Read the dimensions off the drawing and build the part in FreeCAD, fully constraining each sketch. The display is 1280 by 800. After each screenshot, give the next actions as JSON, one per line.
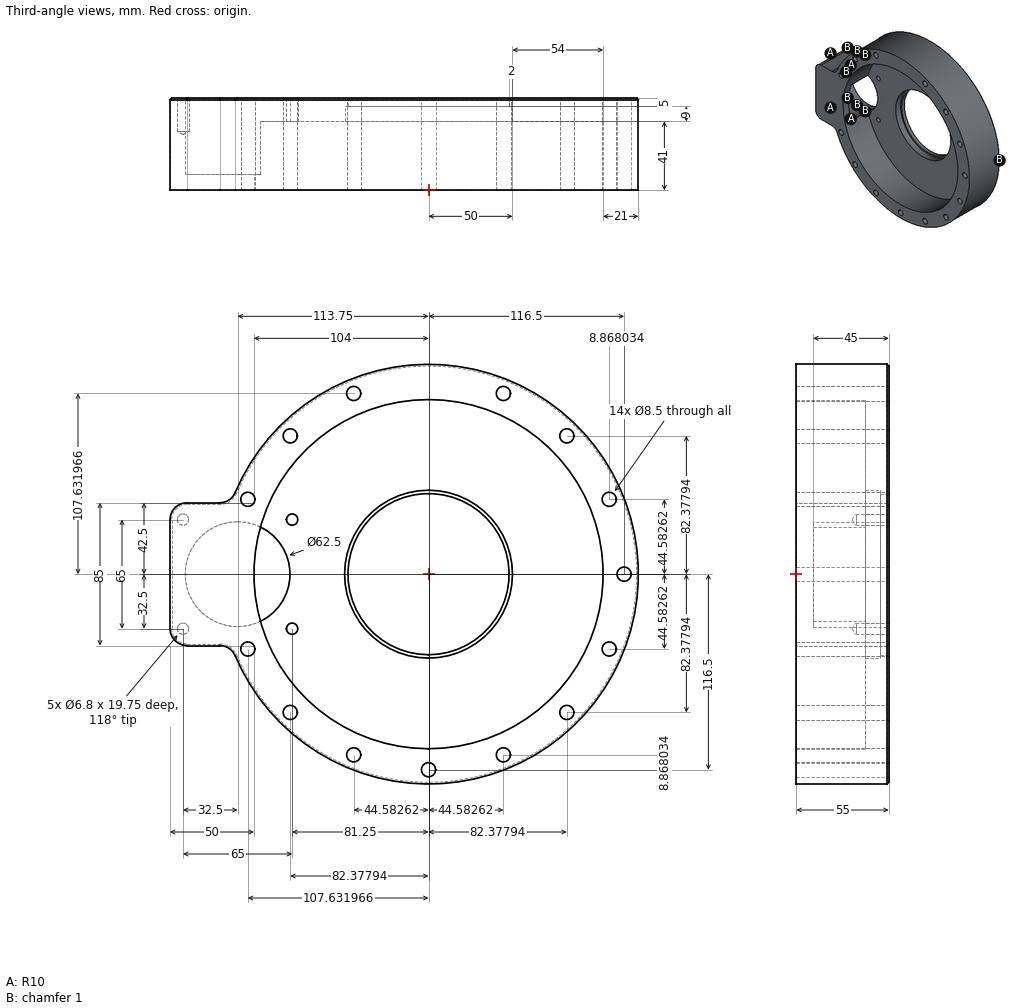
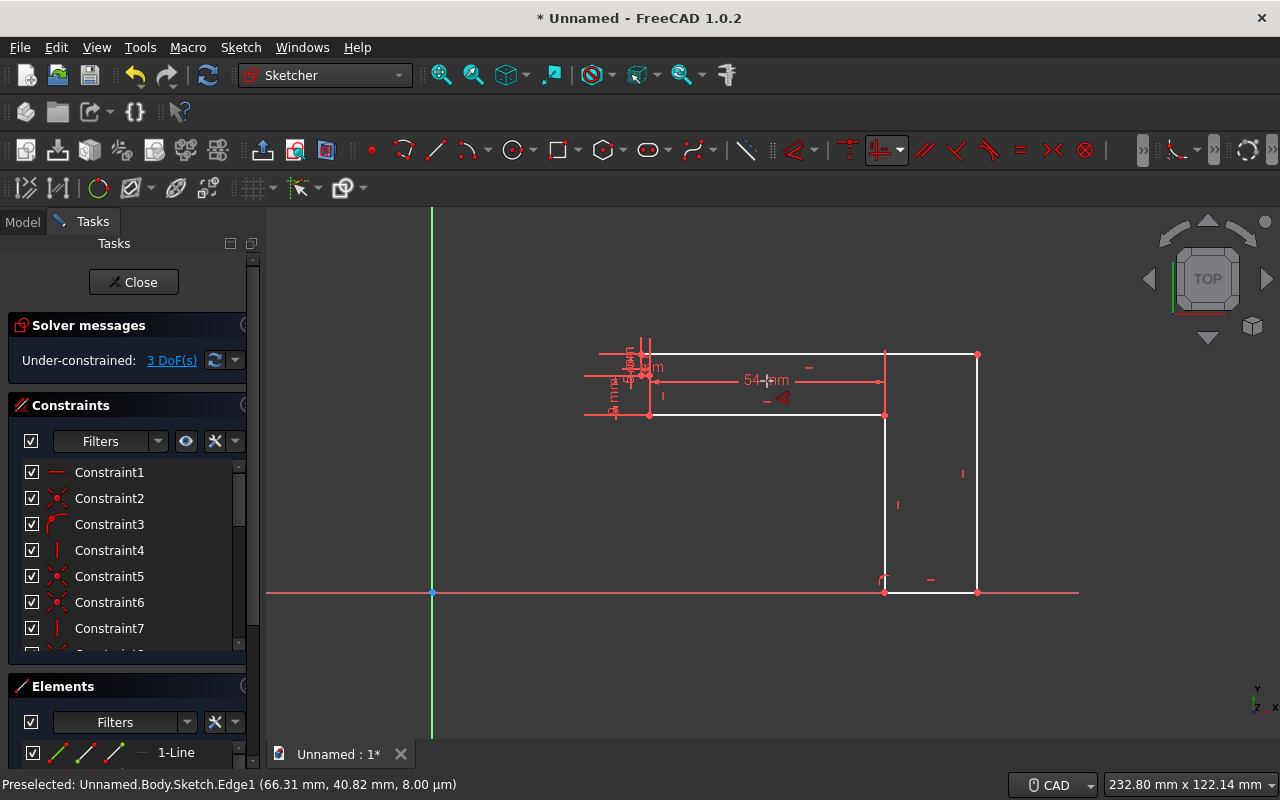
{"action": "left_click", "coordinate": [885, 468]}
{"action": "left_click", "coordinate": [919, 504]}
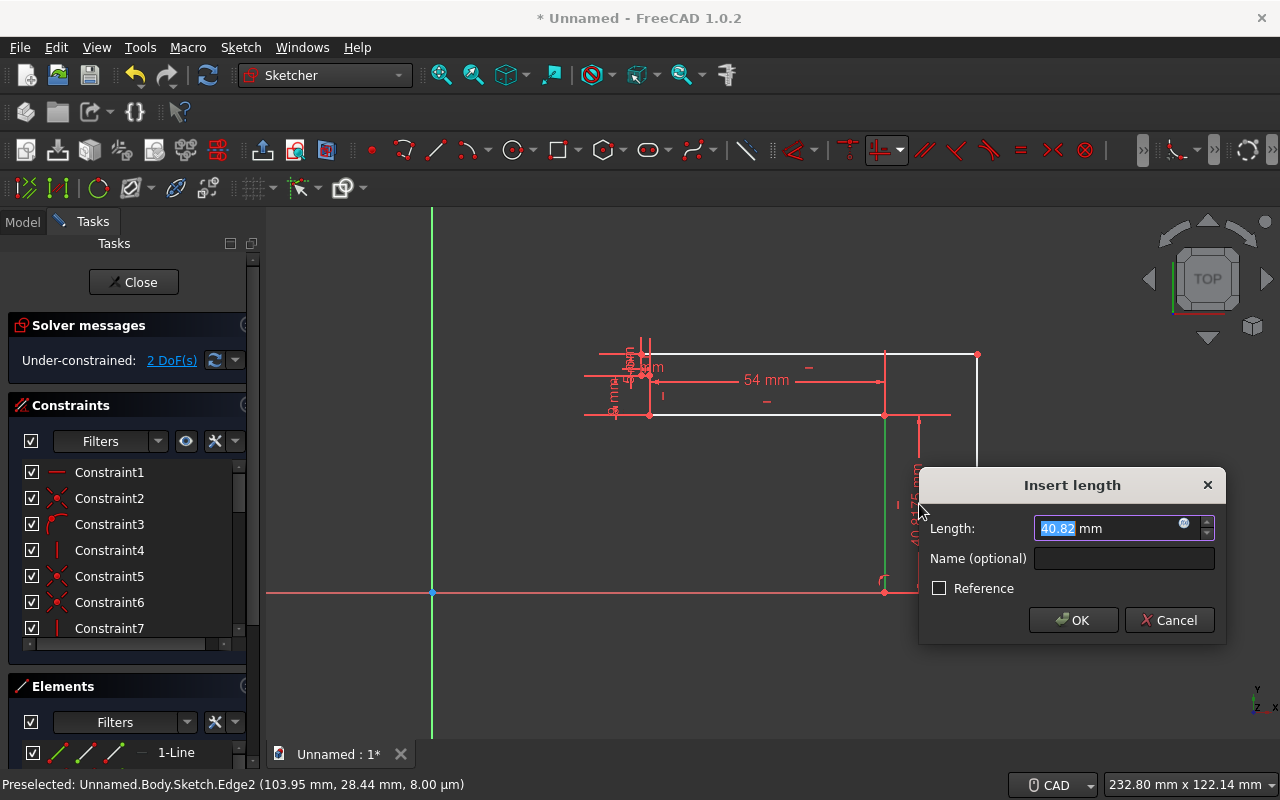
{"action": "type", "text": "41"}
{"action": "key", "text": "Return"}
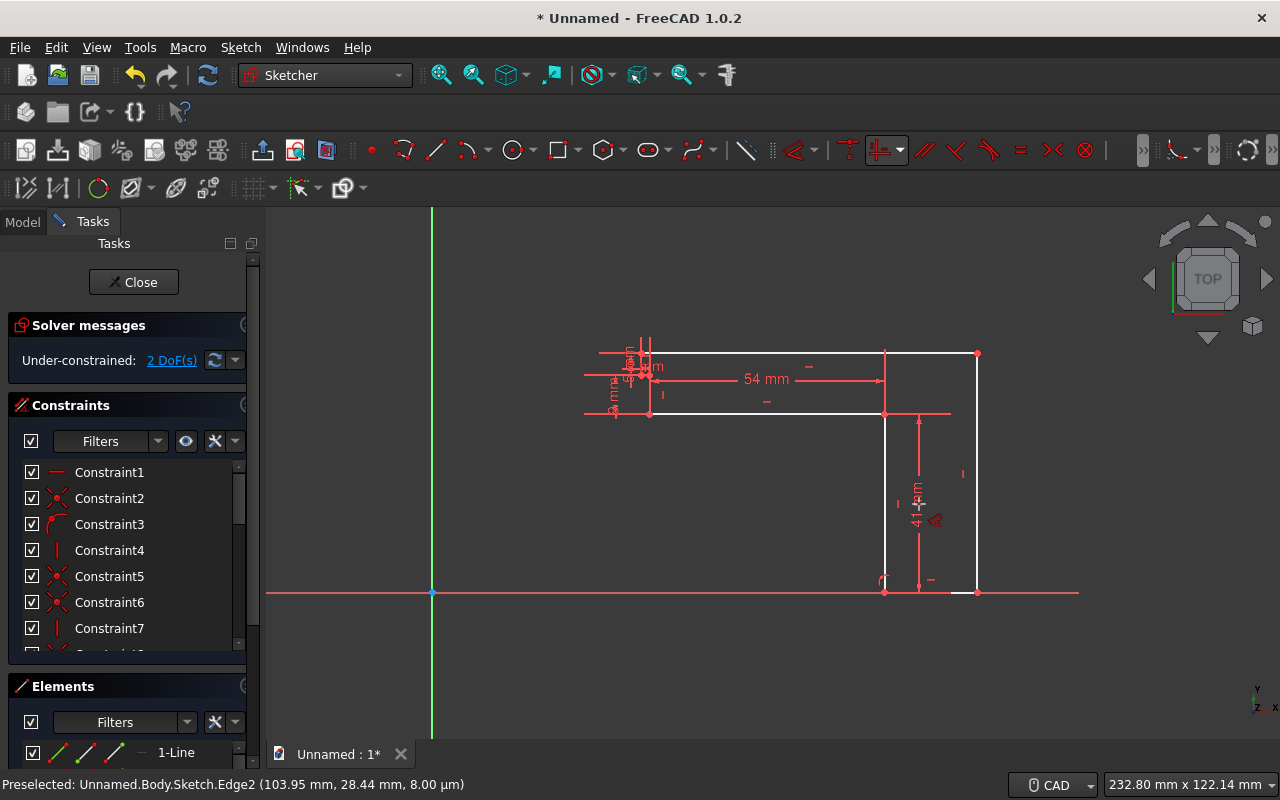
{"action": "left_click", "coordinate": [913, 593]}
{"action": "left_click", "coordinate": [931, 627]}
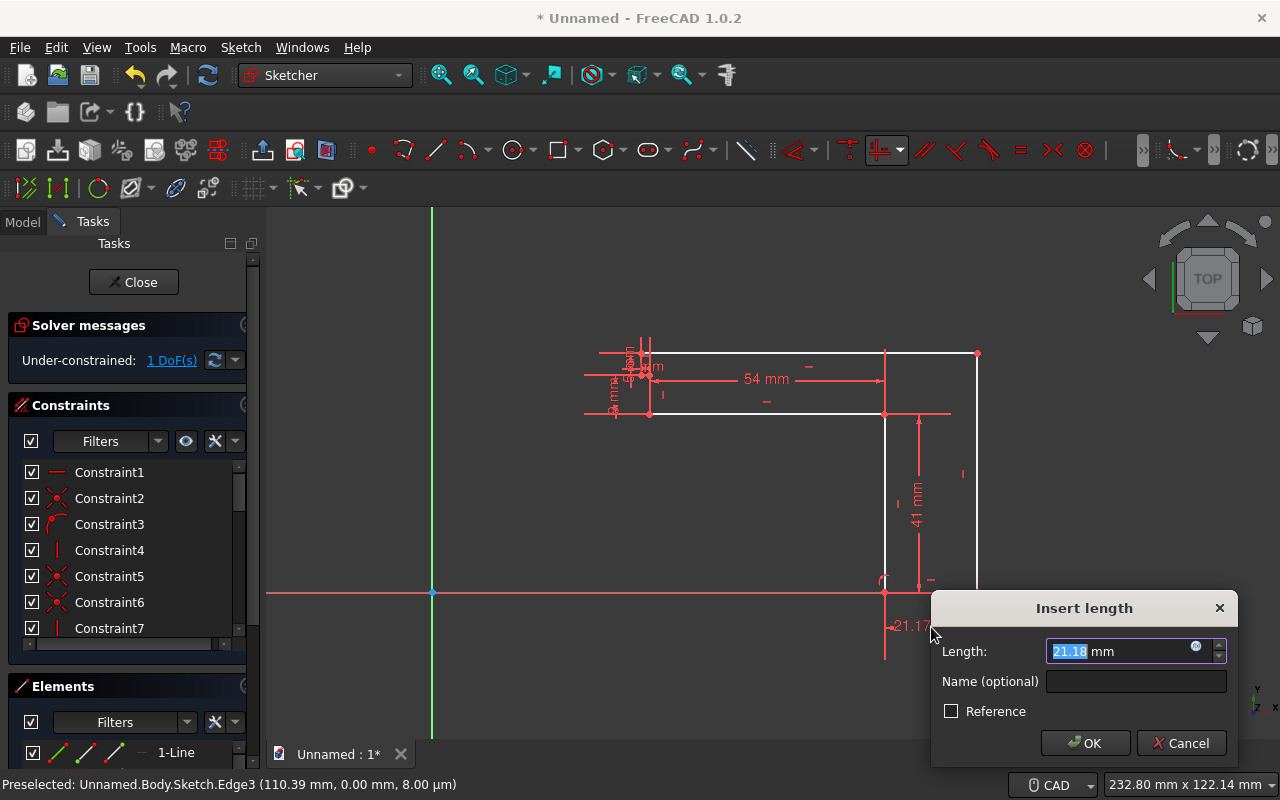
{"action": "type", "text": "21"}
{"action": "key", "text": "Return"}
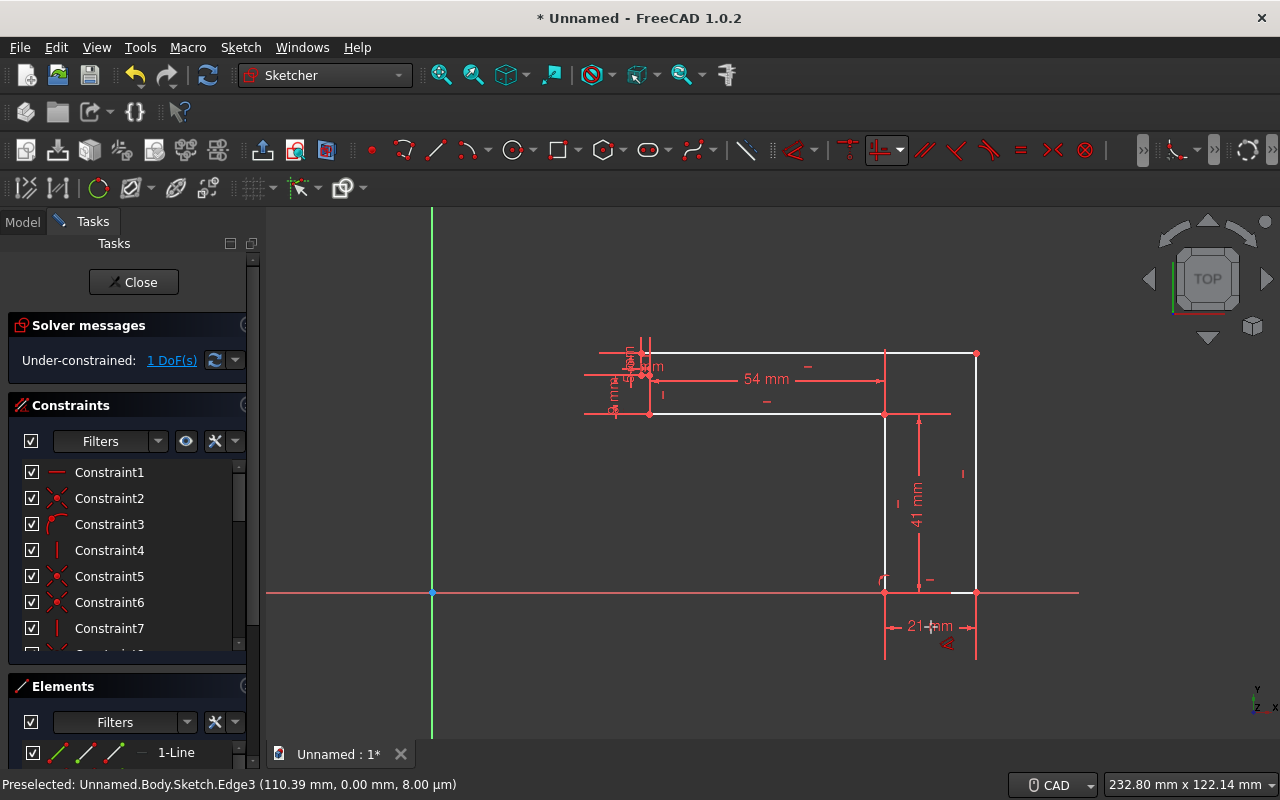
{"action": "left_click", "coordinate": [650, 414]}
{"action": "left_click", "coordinate": [541, 627]}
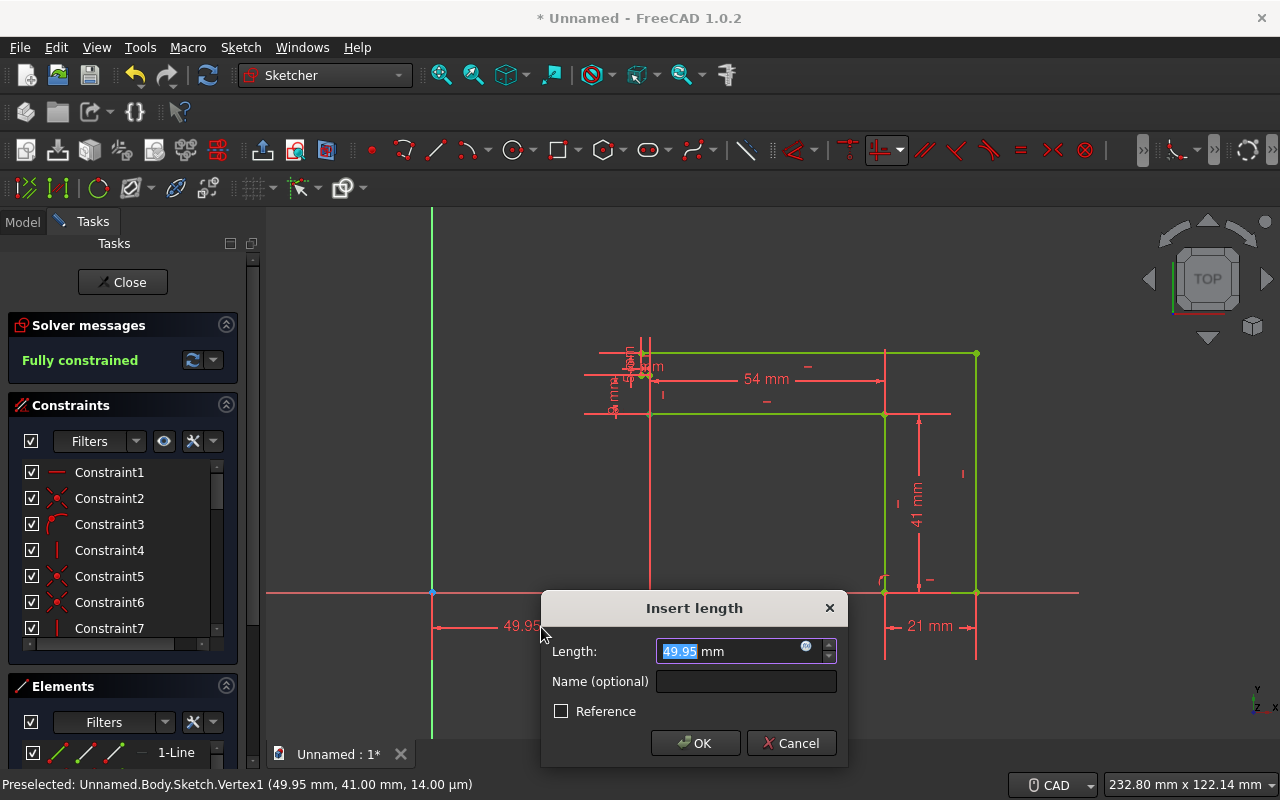
{"action": "type", "text": "50"}
{"action": "key", "text": "Return"}
{"action": "key", "text": "Escape"}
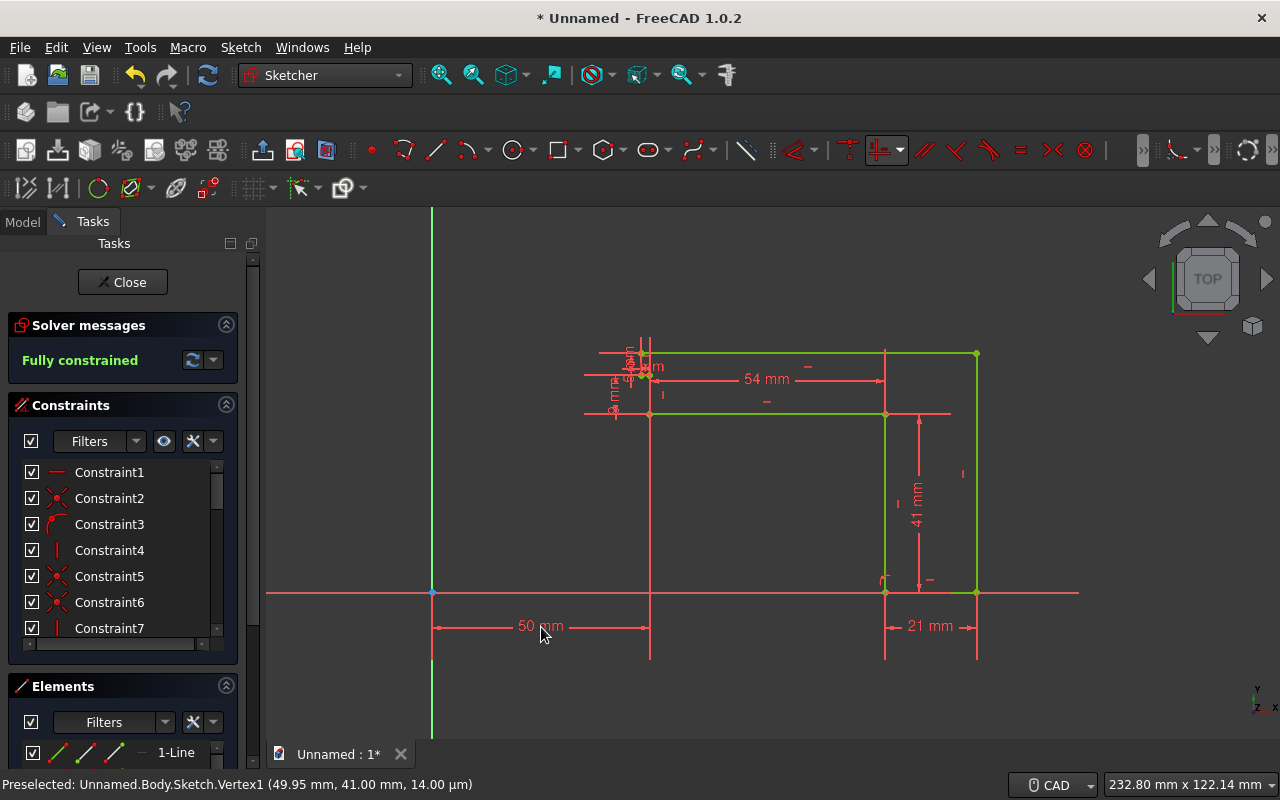
{"action": "left_click", "coordinate": [123, 282]}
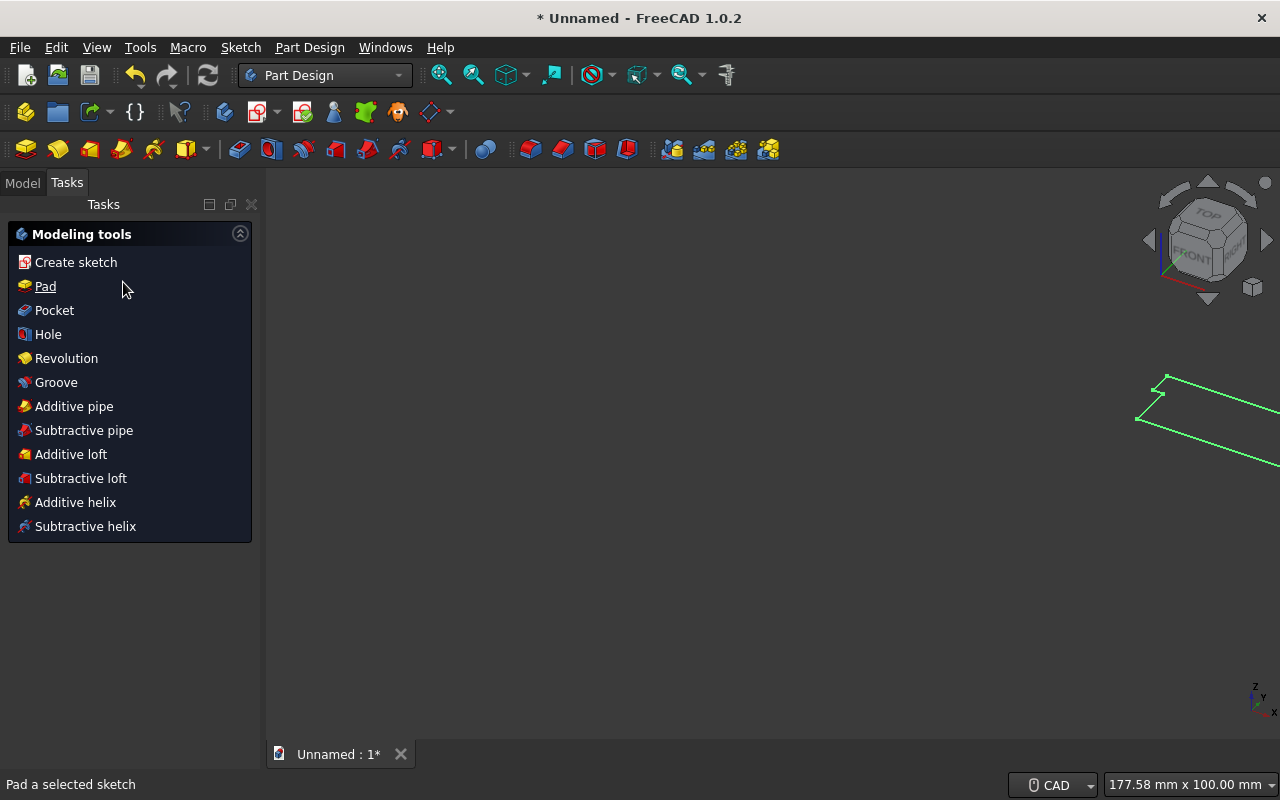
{"action": "left_click", "coordinate": [58, 150]}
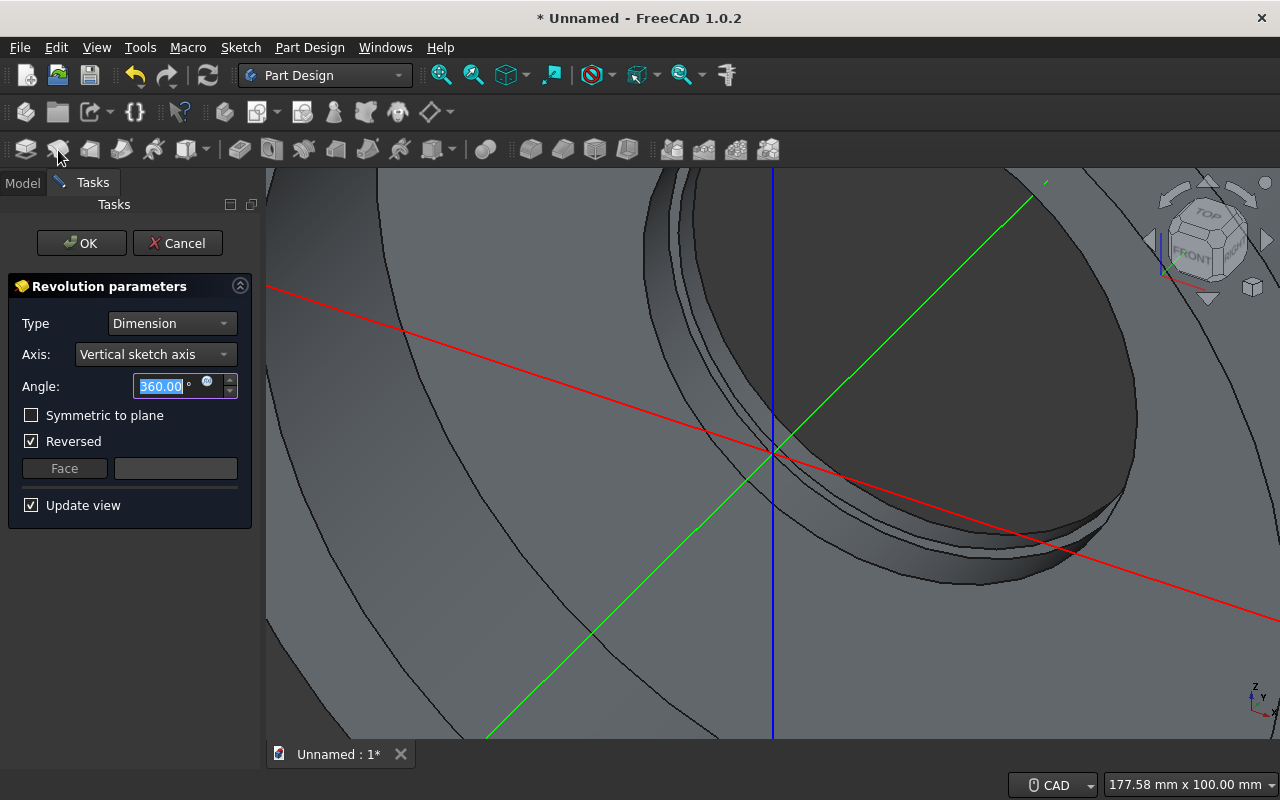
{"action": "left_click", "coordinate": [82, 243]}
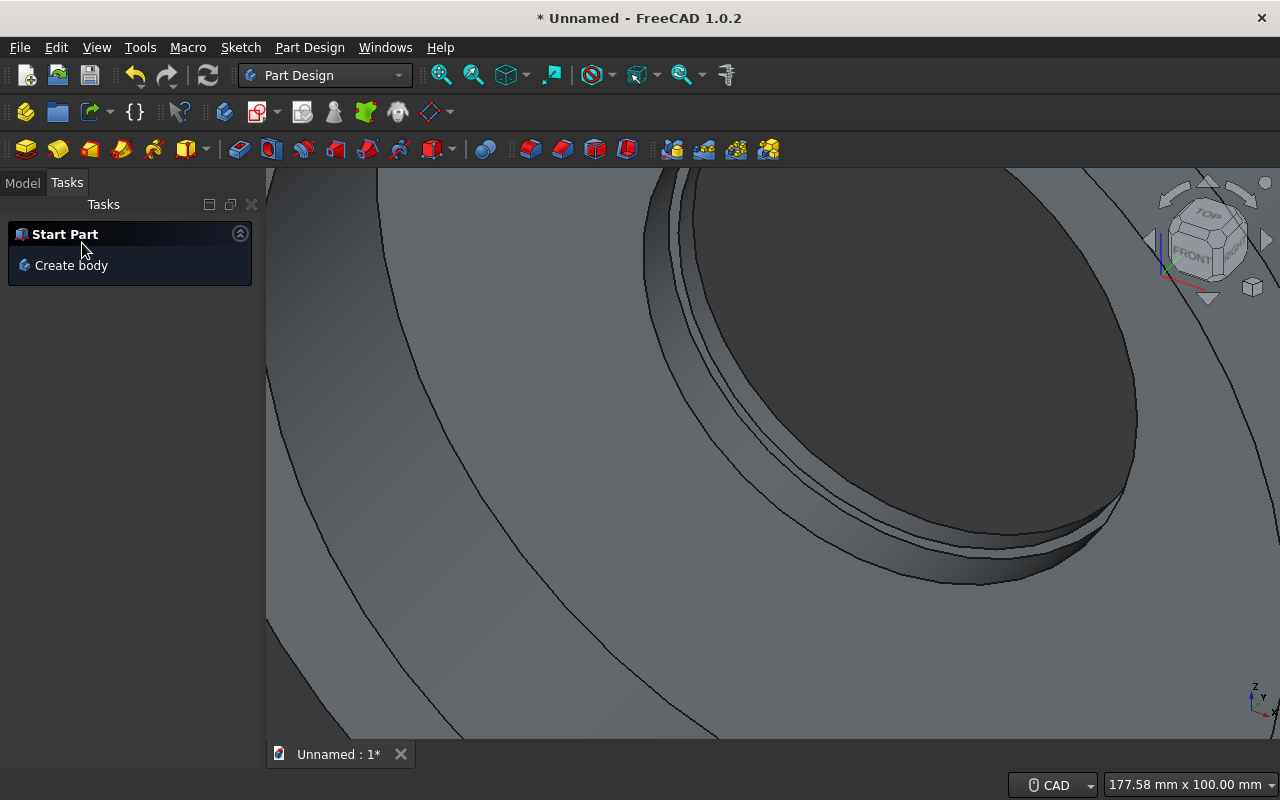
{"action": "left_click", "coordinate": [442, 76]}